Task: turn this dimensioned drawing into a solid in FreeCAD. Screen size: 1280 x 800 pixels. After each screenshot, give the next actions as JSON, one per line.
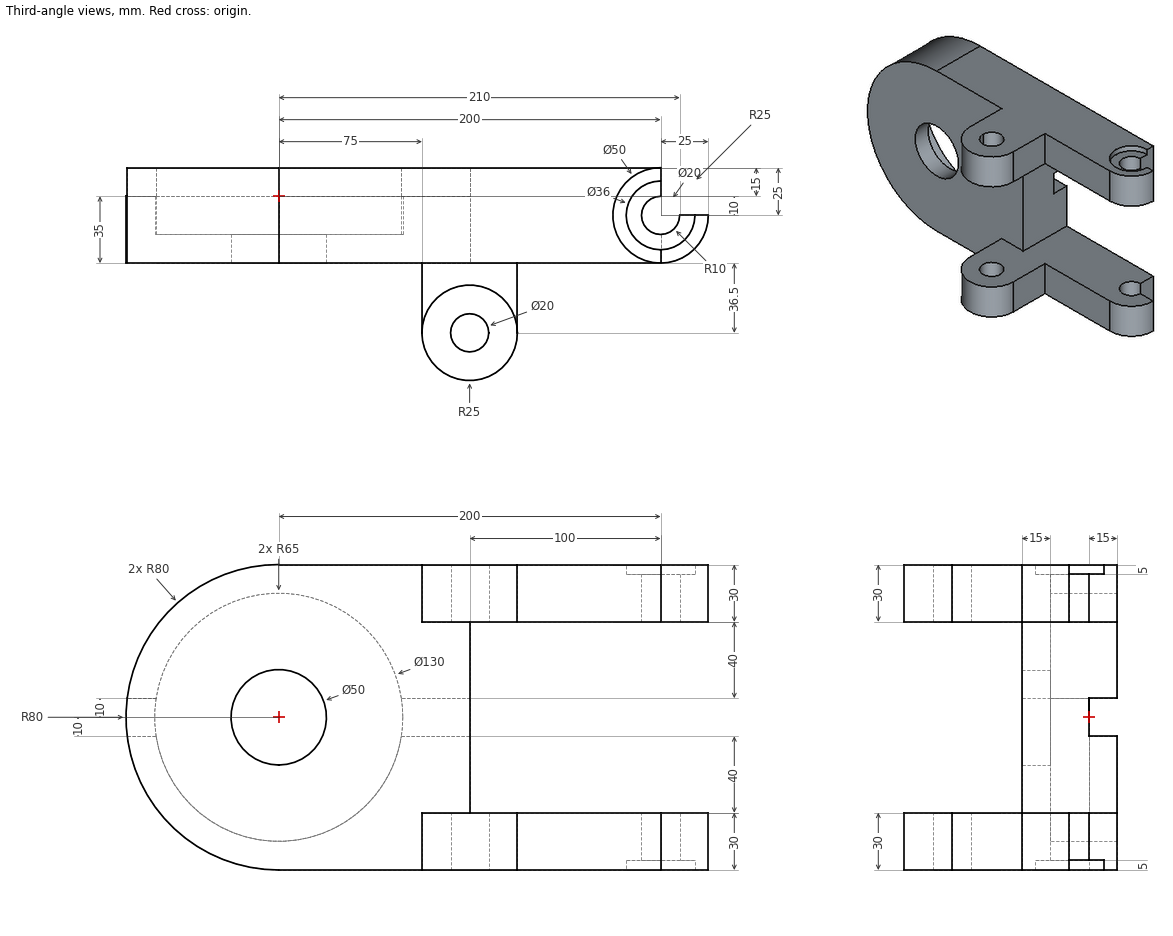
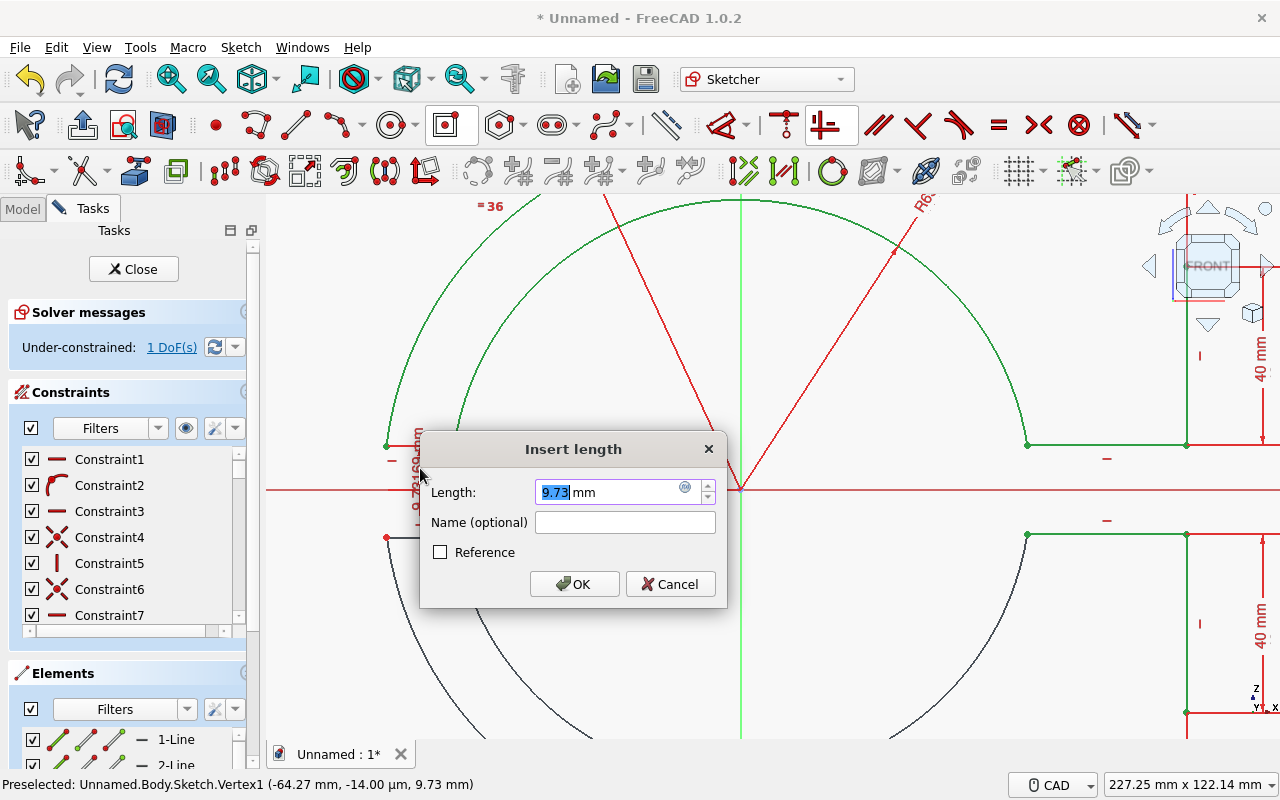
{"action": "type", "text": "10"}
{"action": "key", "text": "Return"}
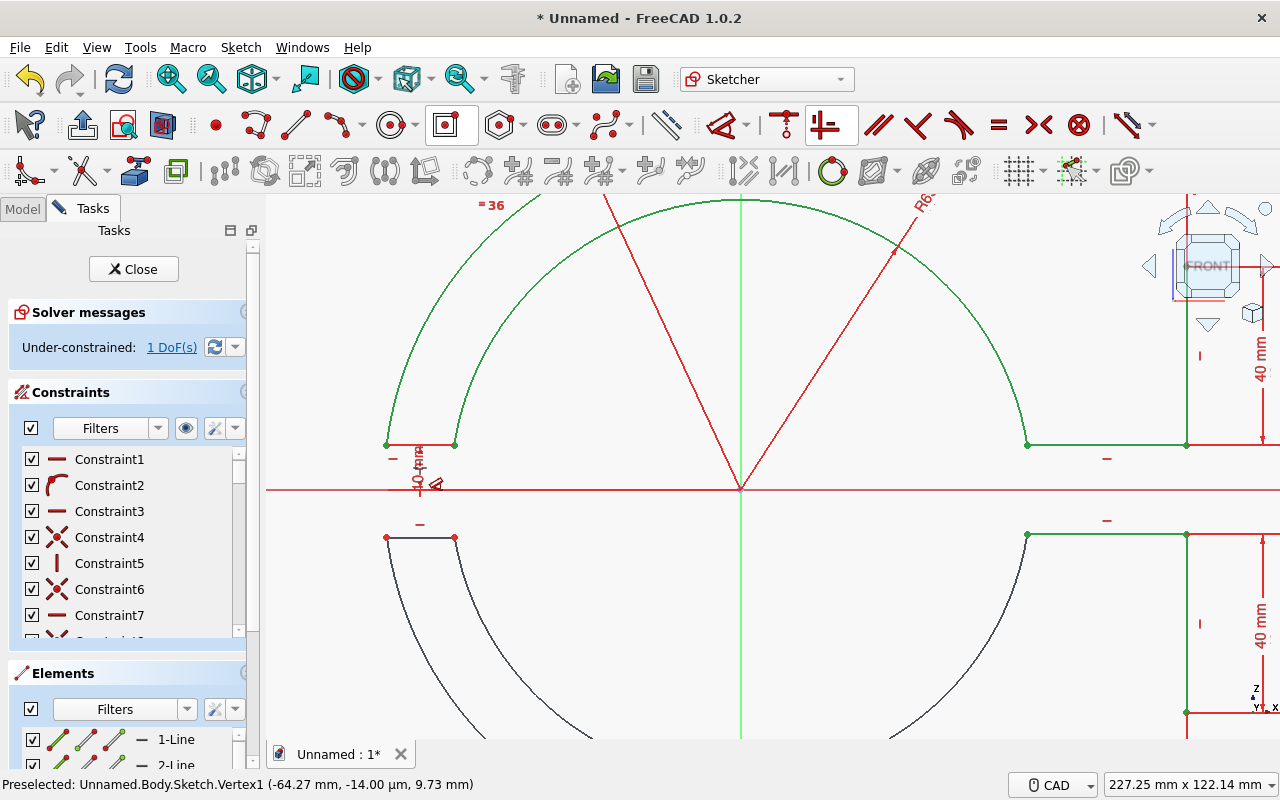
{"action": "left_click", "coordinate": [387, 538]}
{"action": "left_click", "coordinate": [353, 514]}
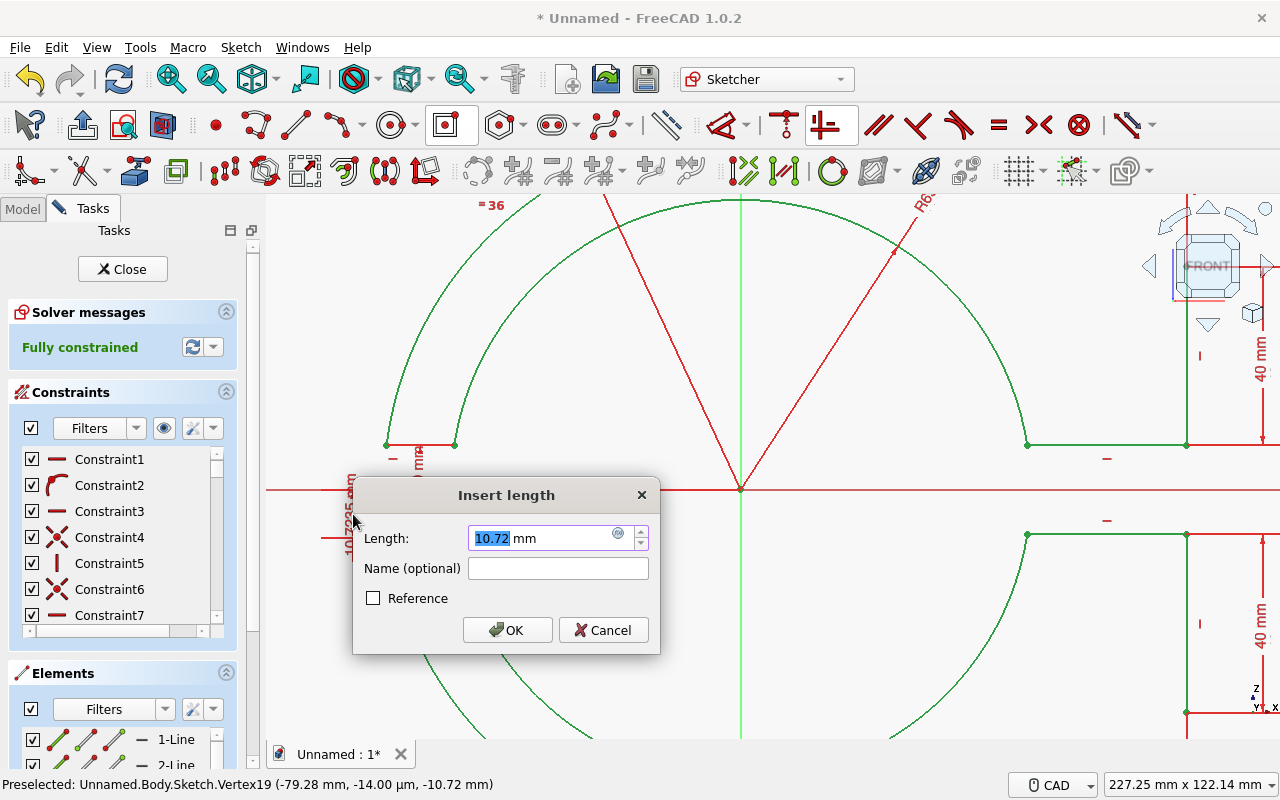
{"action": "type", "text": "10"}
{"action": "key", "text": "Return"}
{"action": "key", "text": "Escape"}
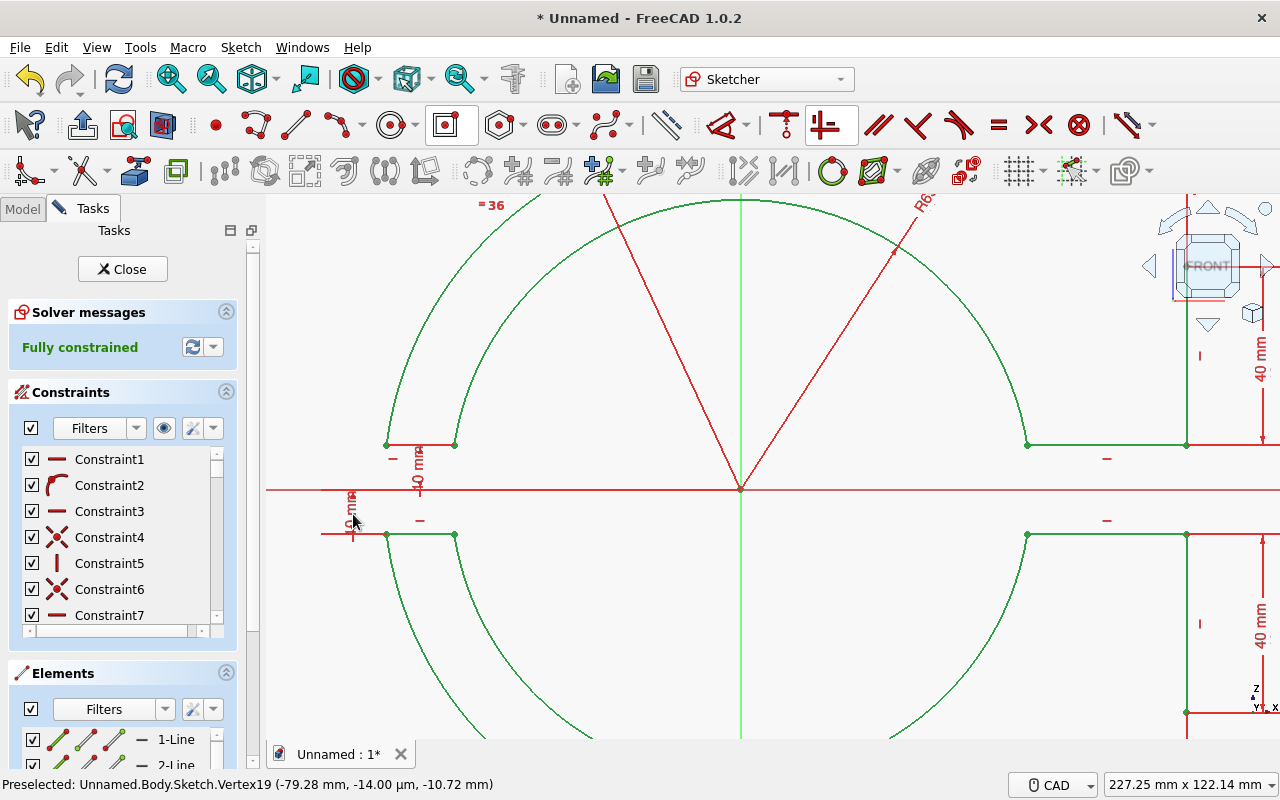
{"action": "left_click", "coordinate": [123, 269]}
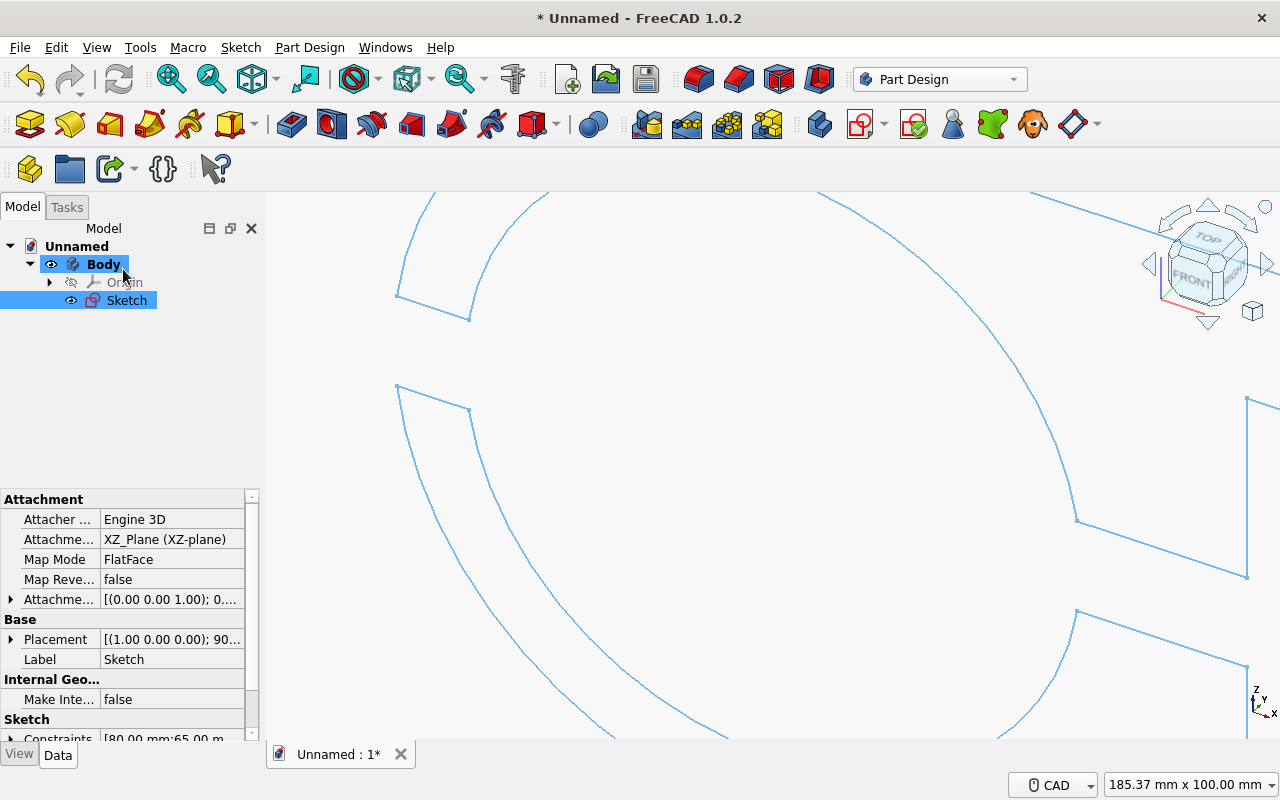
{"action": "left_click", "coordinate": [30, 124]}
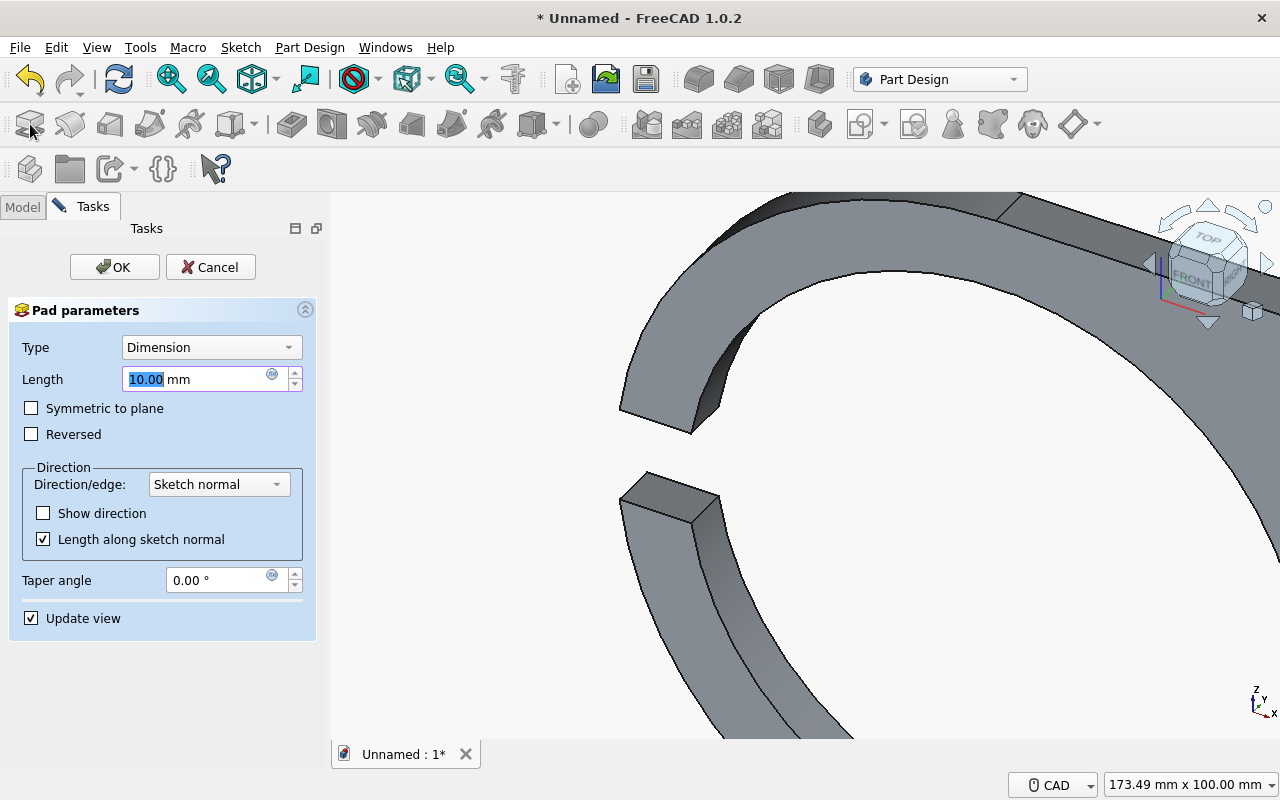
{"action": "type", "text": "15"}
{"action": "key", "text": "Tab"}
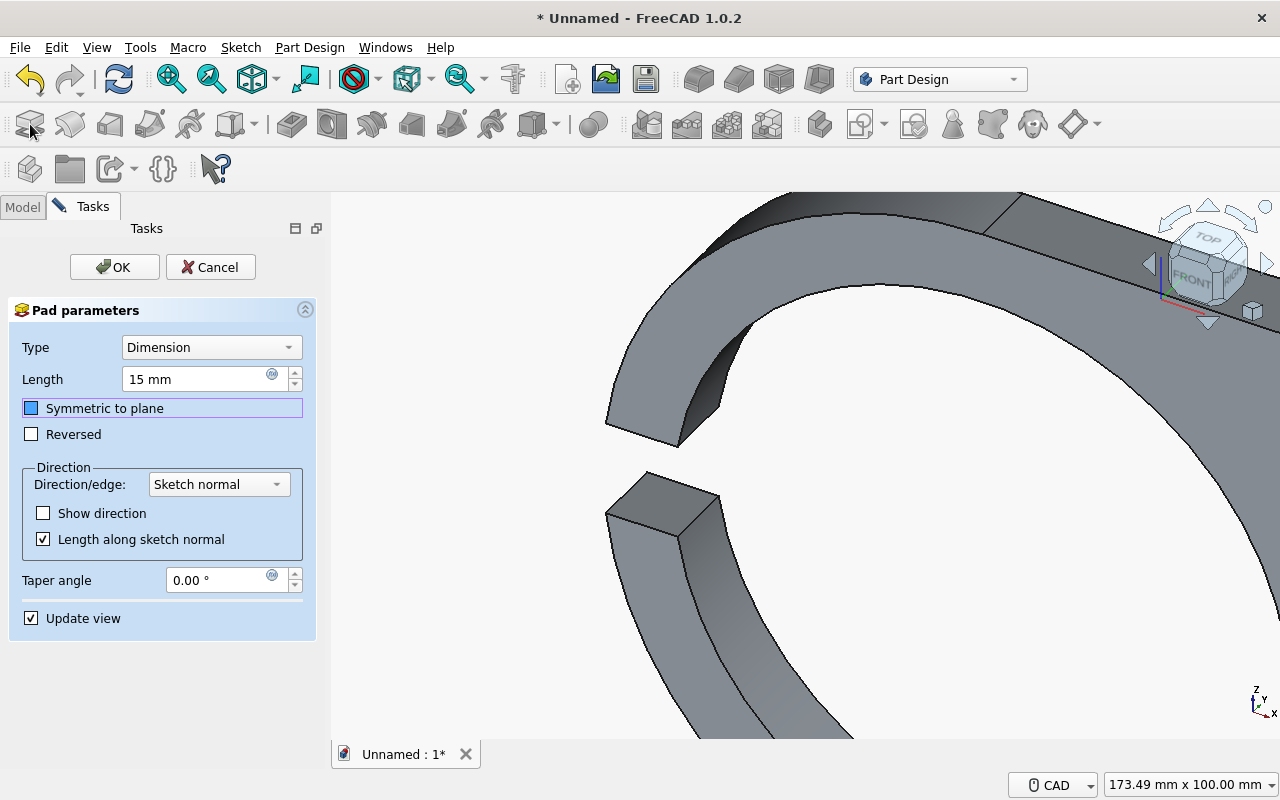
{"action": "left_click", "coordinate": [30, 434]}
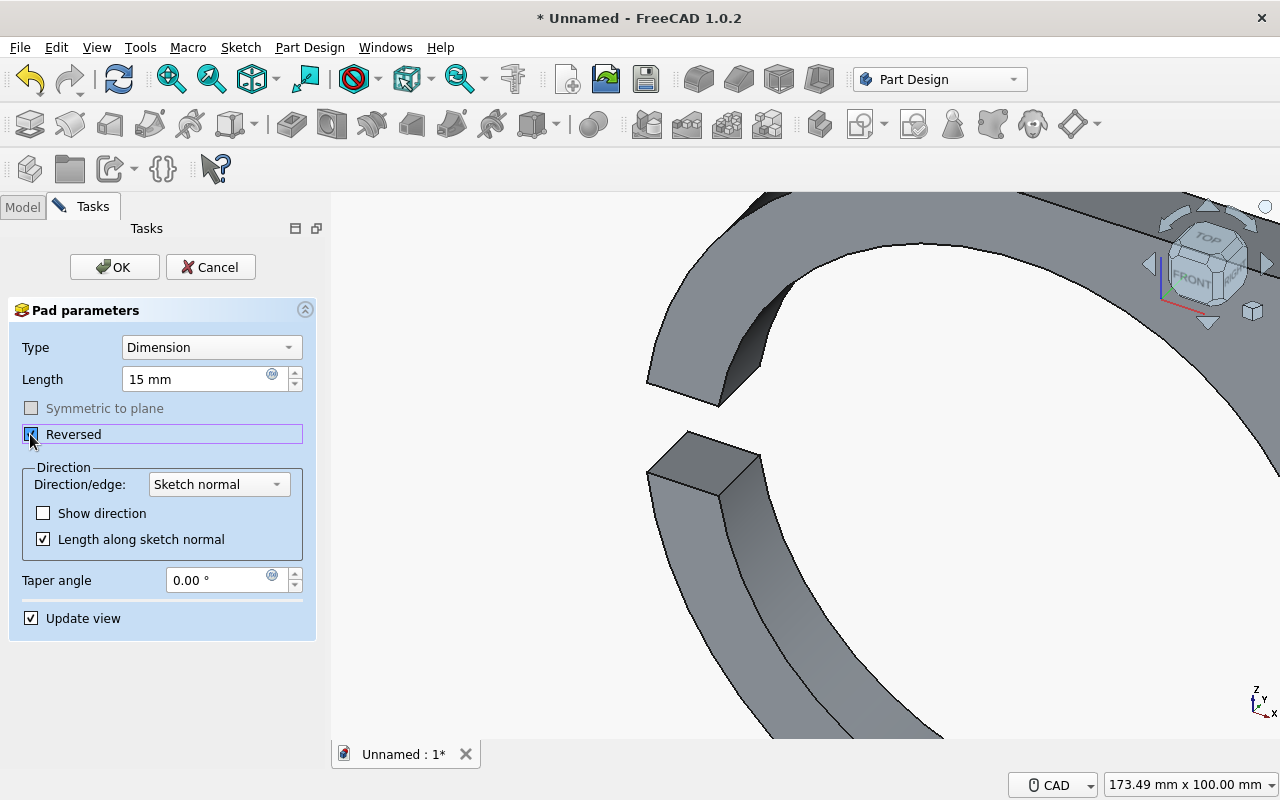
{"action": "left_click", "coordinate": [115, 267]}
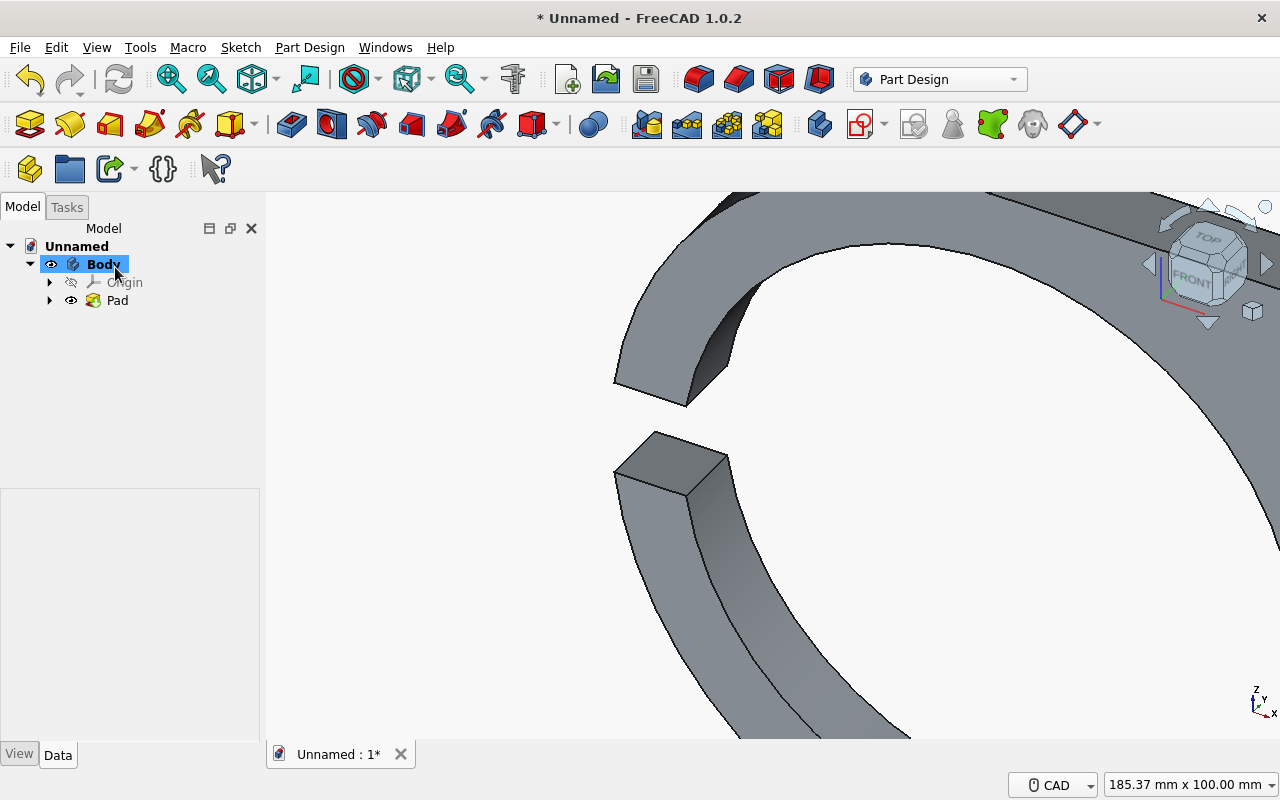
{"action": "left_click", "coordinate": [172, 80]}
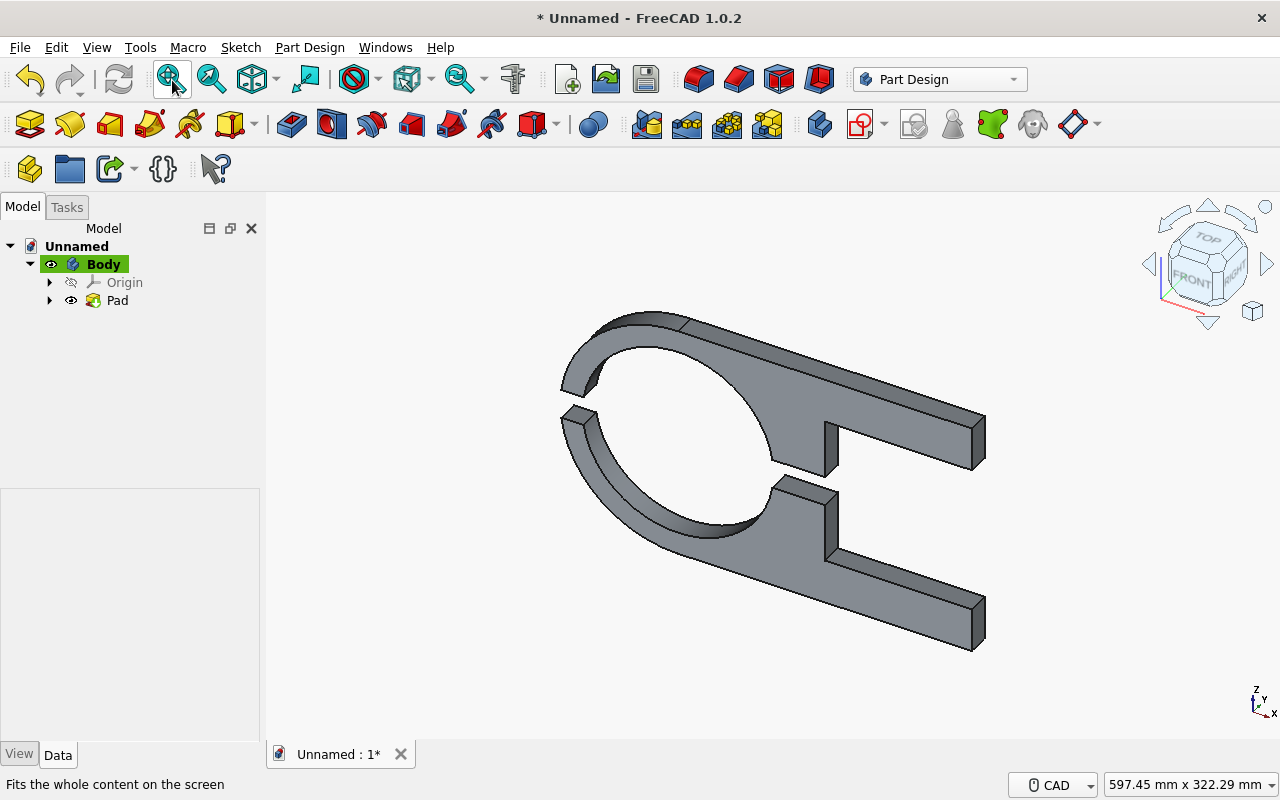
{"action": "left_click", "coordinate": [50, 282]}